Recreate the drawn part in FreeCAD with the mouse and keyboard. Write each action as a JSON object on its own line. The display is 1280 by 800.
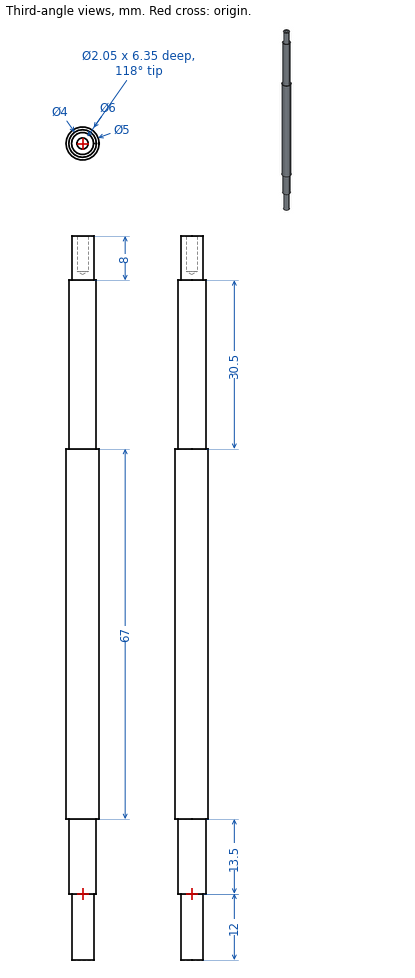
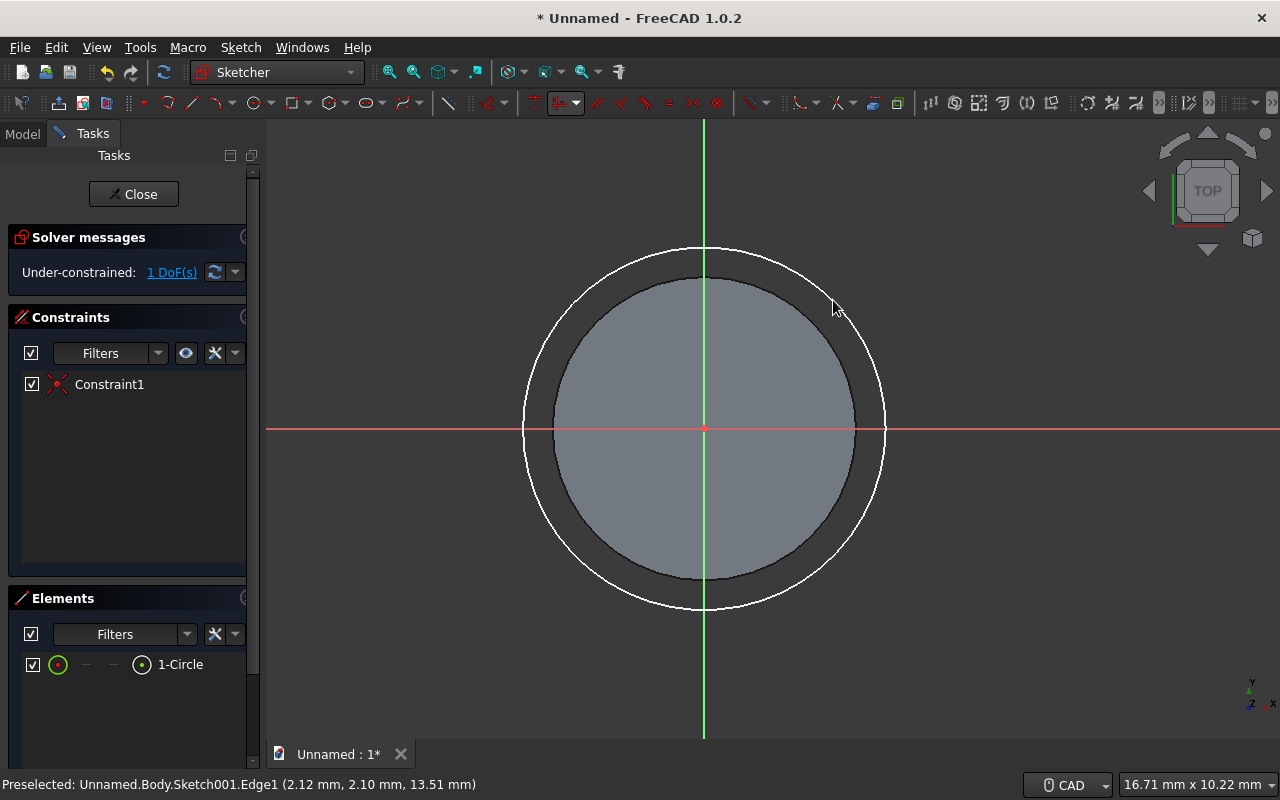
{"action": "left_click", "coordinate": [488, 104]}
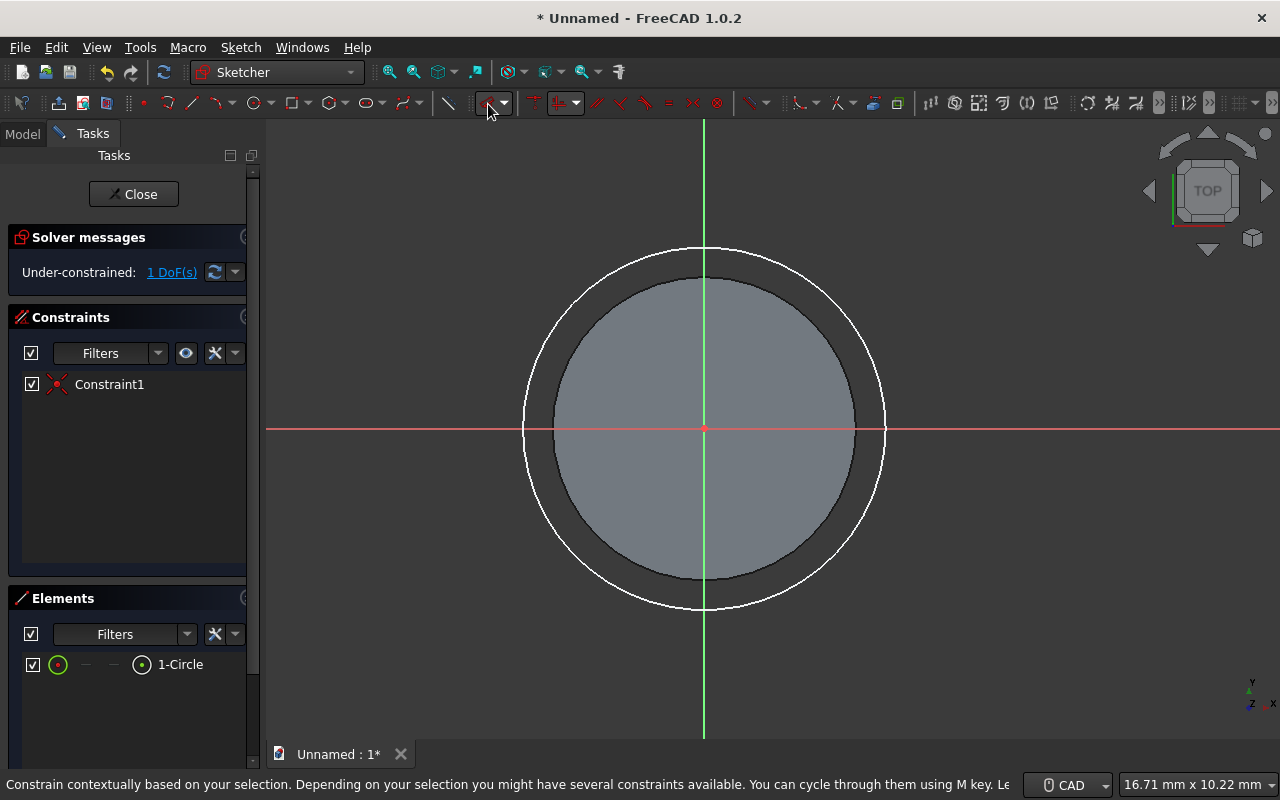
{"action": "left_click", "coordinate": [832, 300]}
{"action": "left_click", "coordinate": [855, 277]}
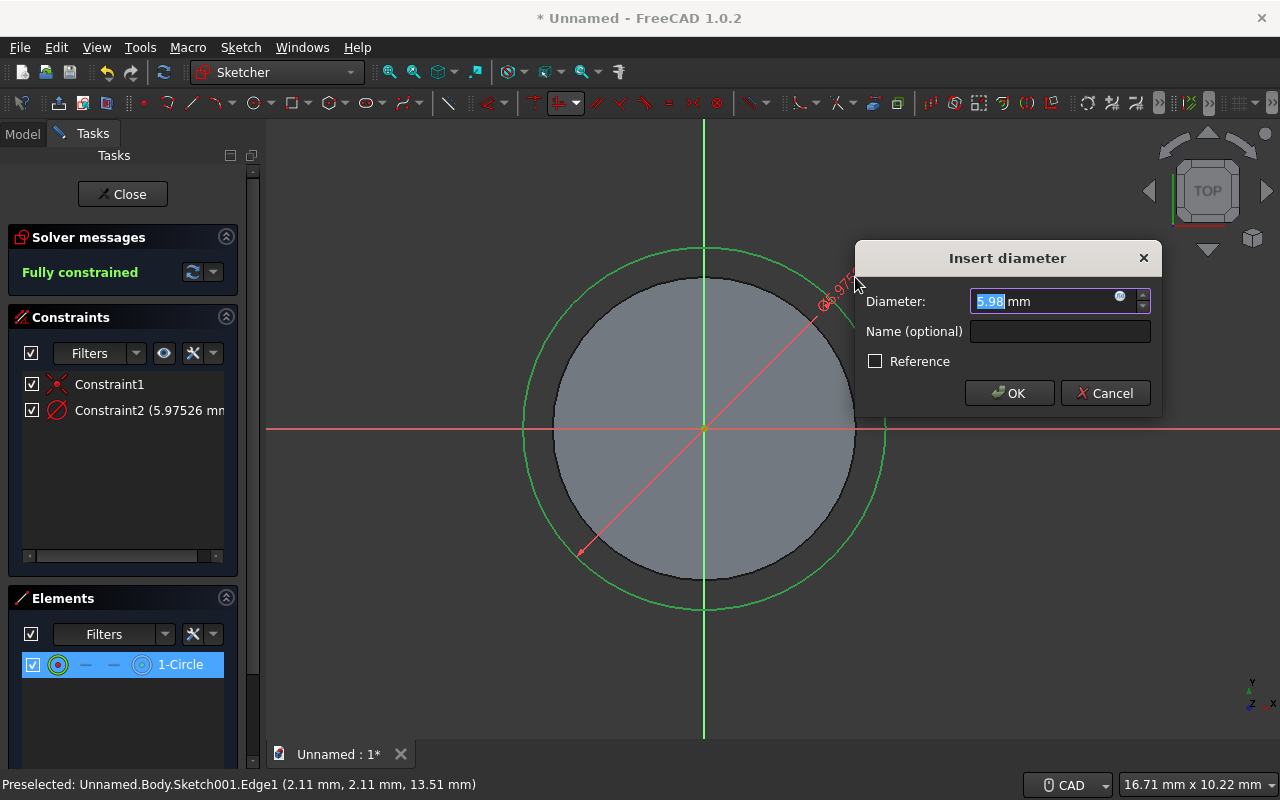
{"action": "type", "text": "6"}
{"action": "key", "text": "Return"}
{"action": "key", "text": "Escape"}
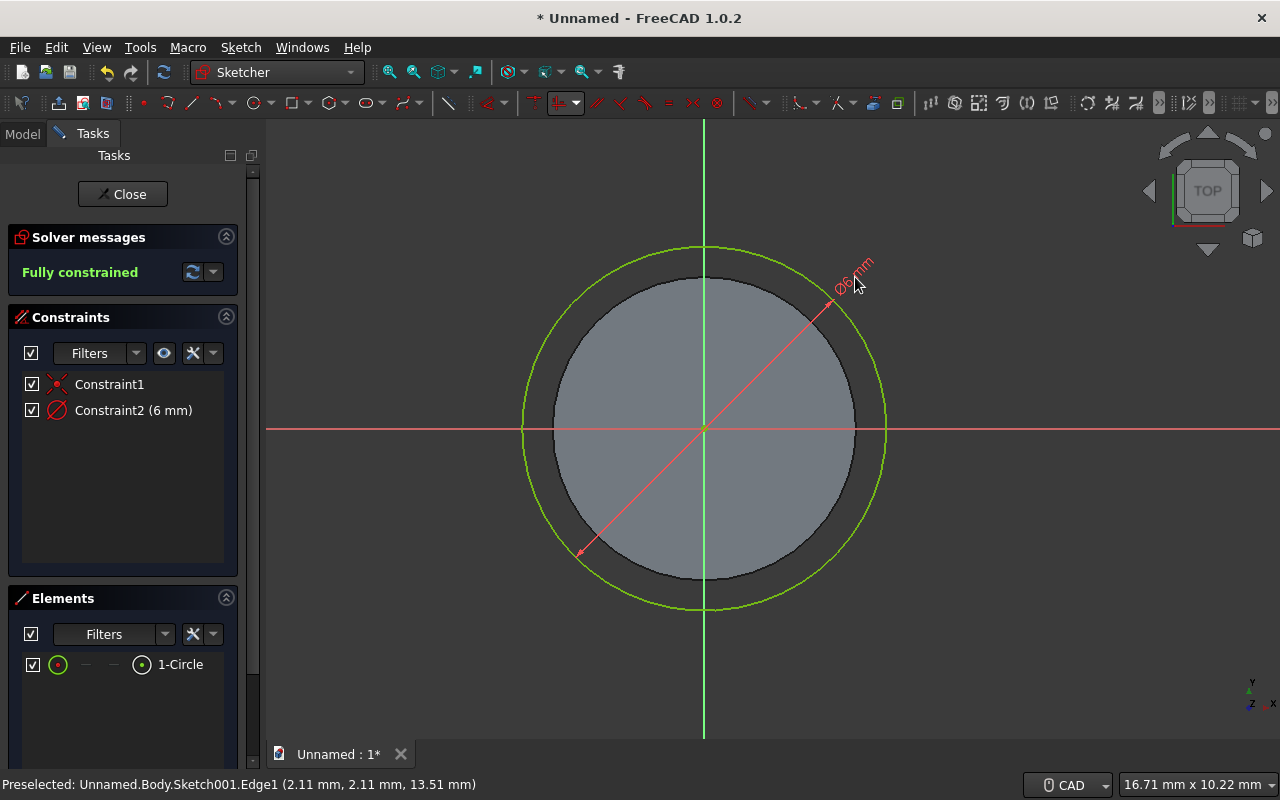
{"action": "left_click", "coordinate": [123, 194]}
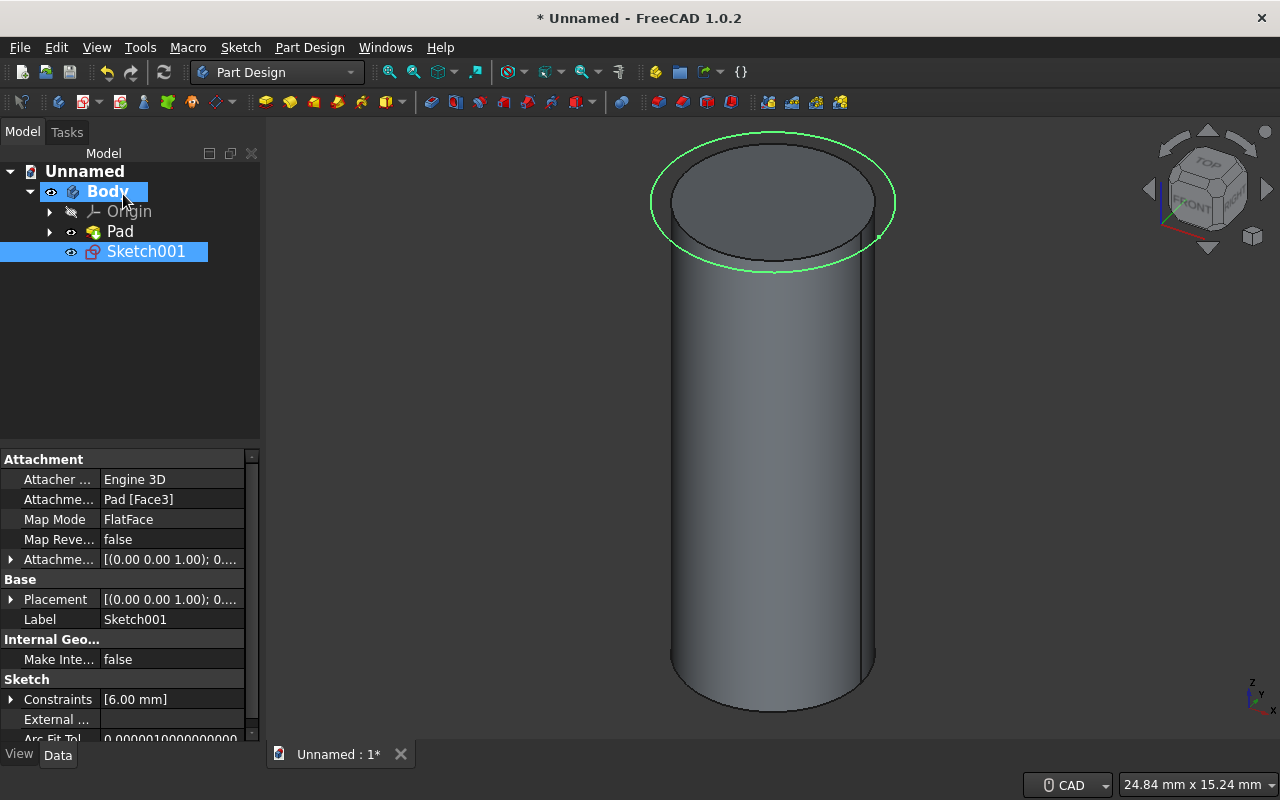
{"action": "left_click", "coordinate": [266, 102]}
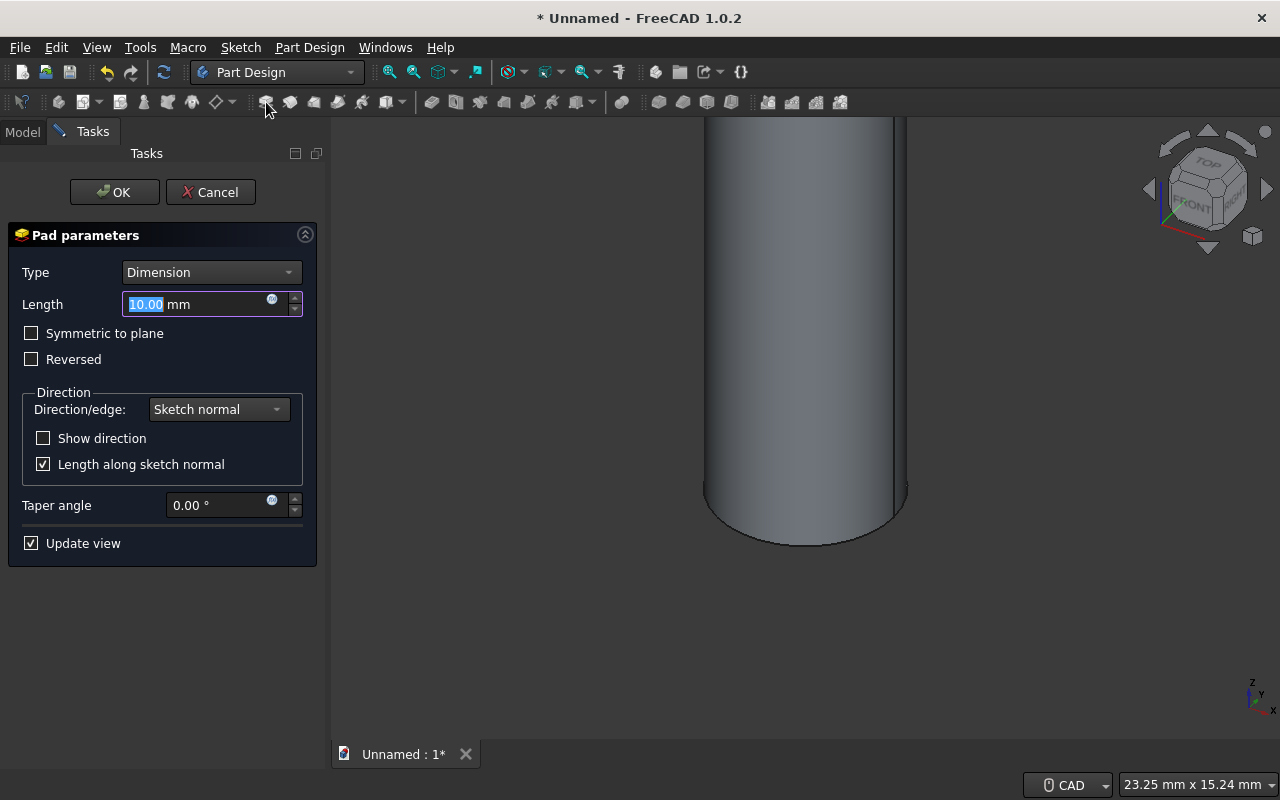
{"action": "type", "text": "67"}
{"action": "key", "text": "Tab"}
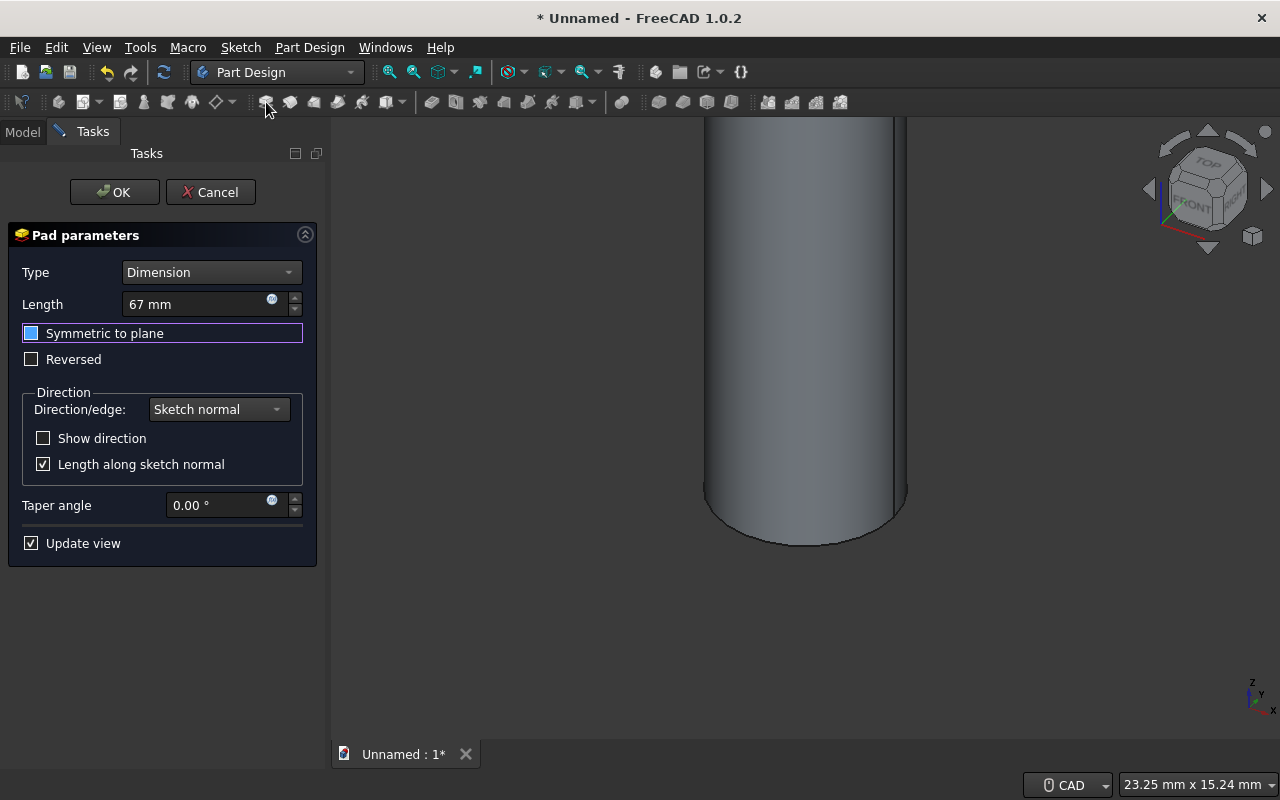
{"action": "left_click", "coordinate": [115, 192]}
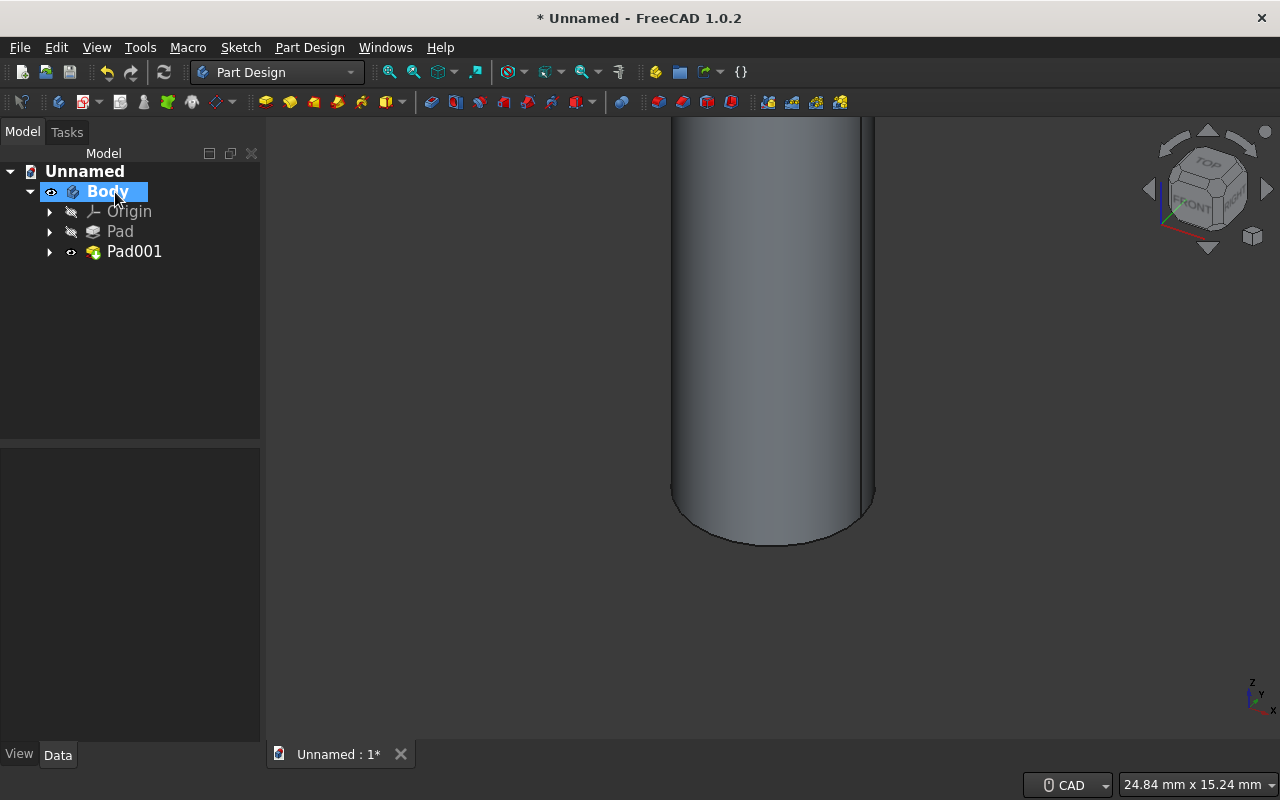
{"action": "left_click", "coordinate": [390, 72]}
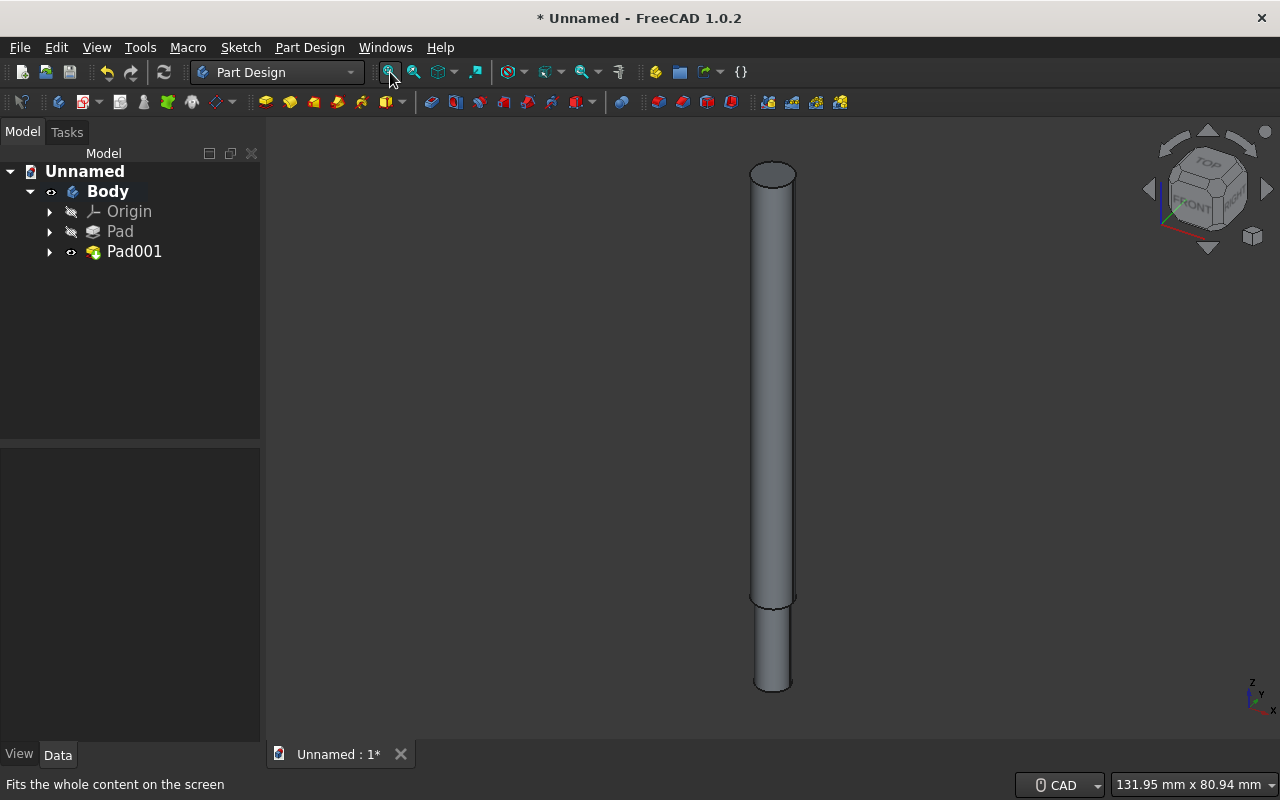
{"action": "left_click", "coordinate": [773, 174]}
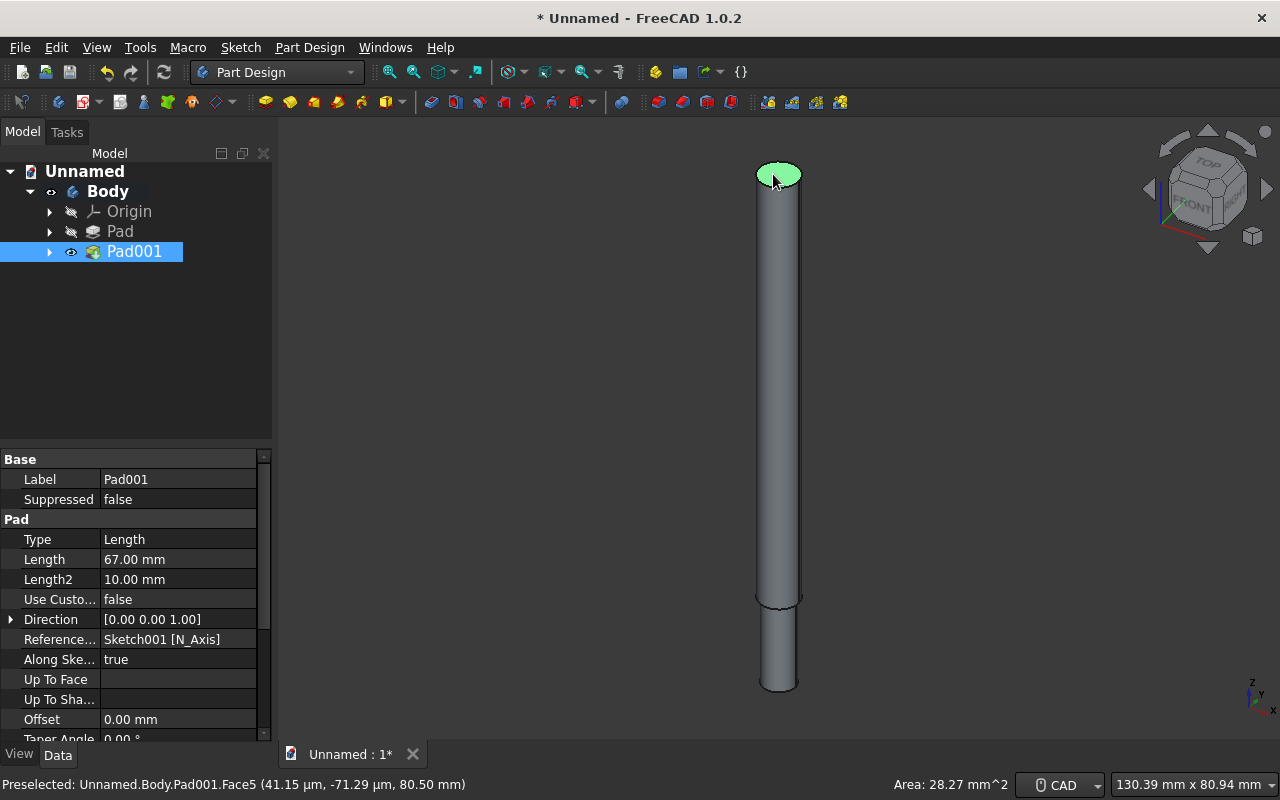
{"action": "left_click", "coordinate": [84, 102]}